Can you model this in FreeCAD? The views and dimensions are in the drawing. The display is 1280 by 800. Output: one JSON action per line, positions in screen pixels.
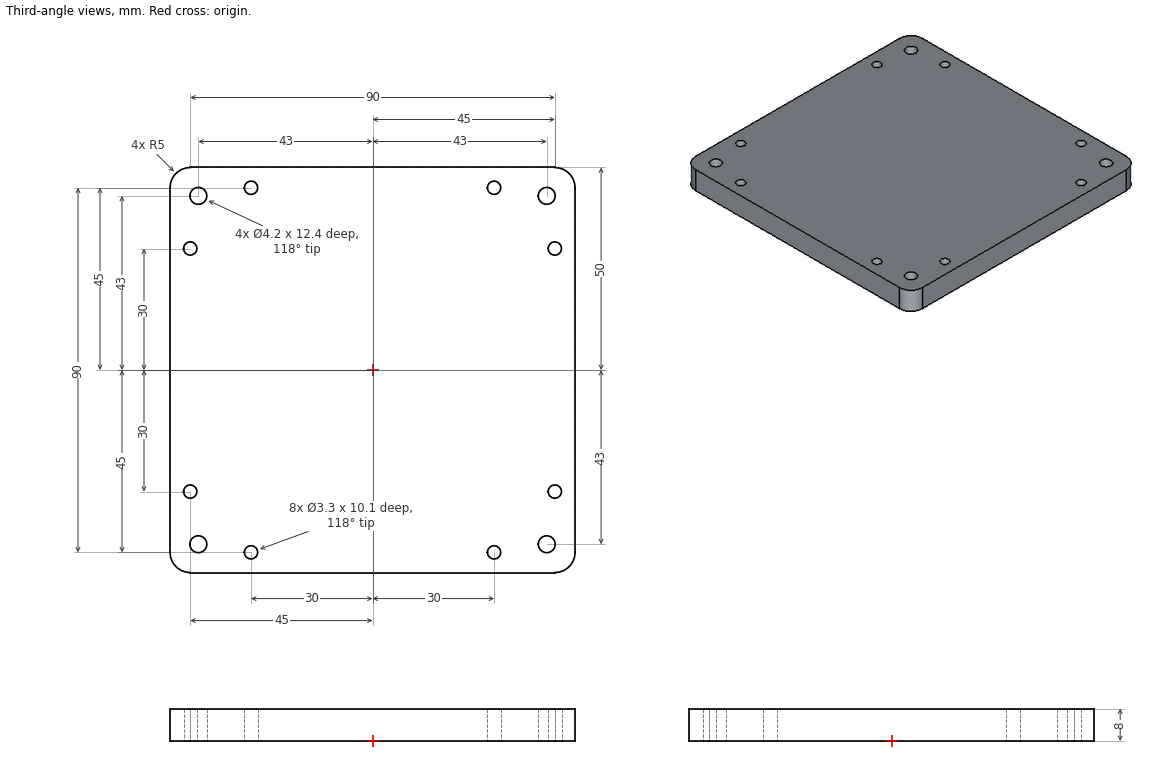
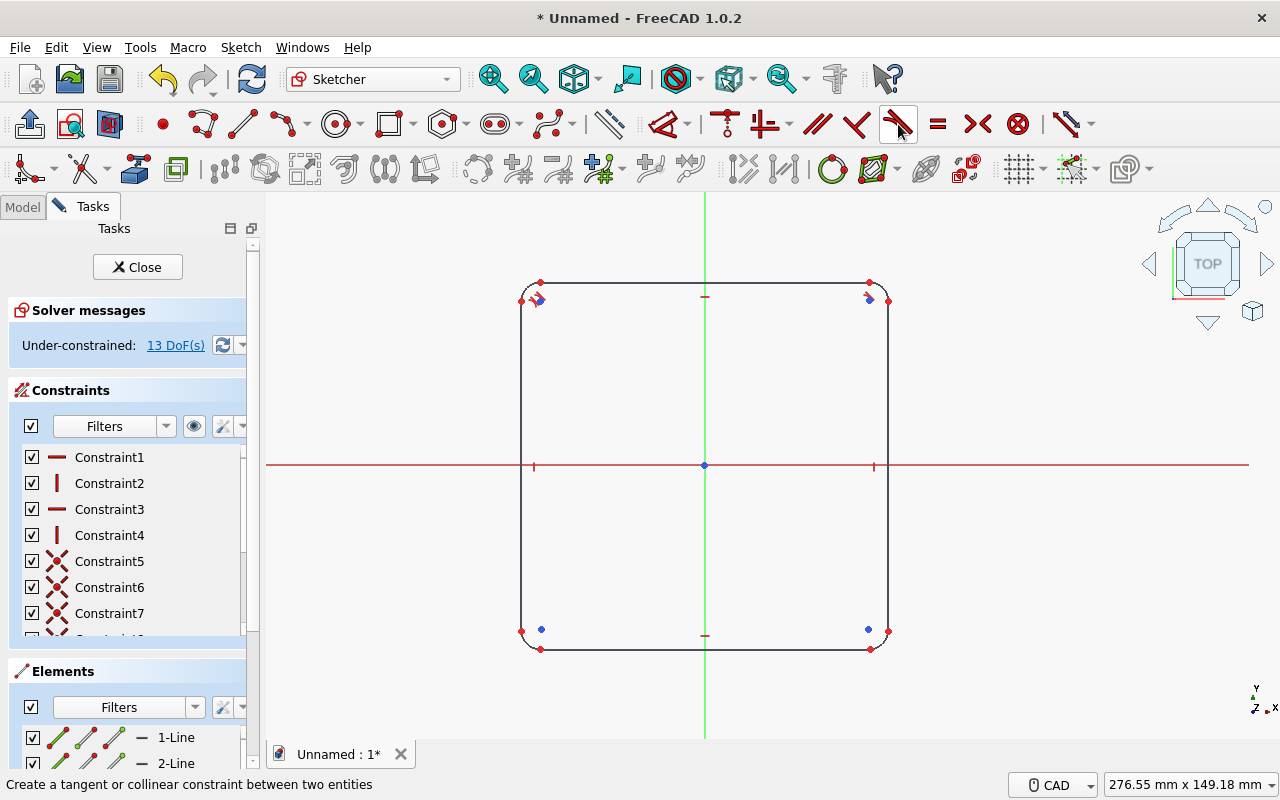
{"action": "left_click", "coordinate": [521, 401]}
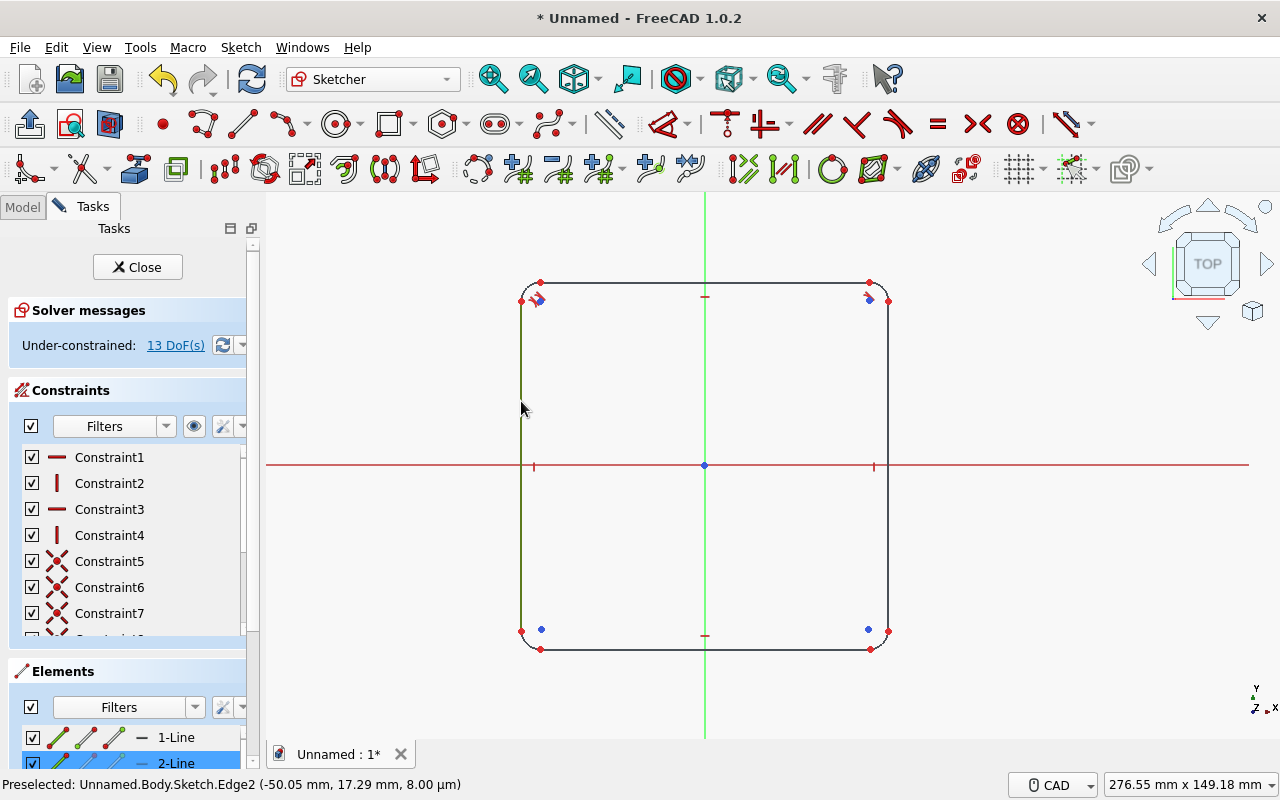
{"action": "left_click", "coordinate": [527, 644]}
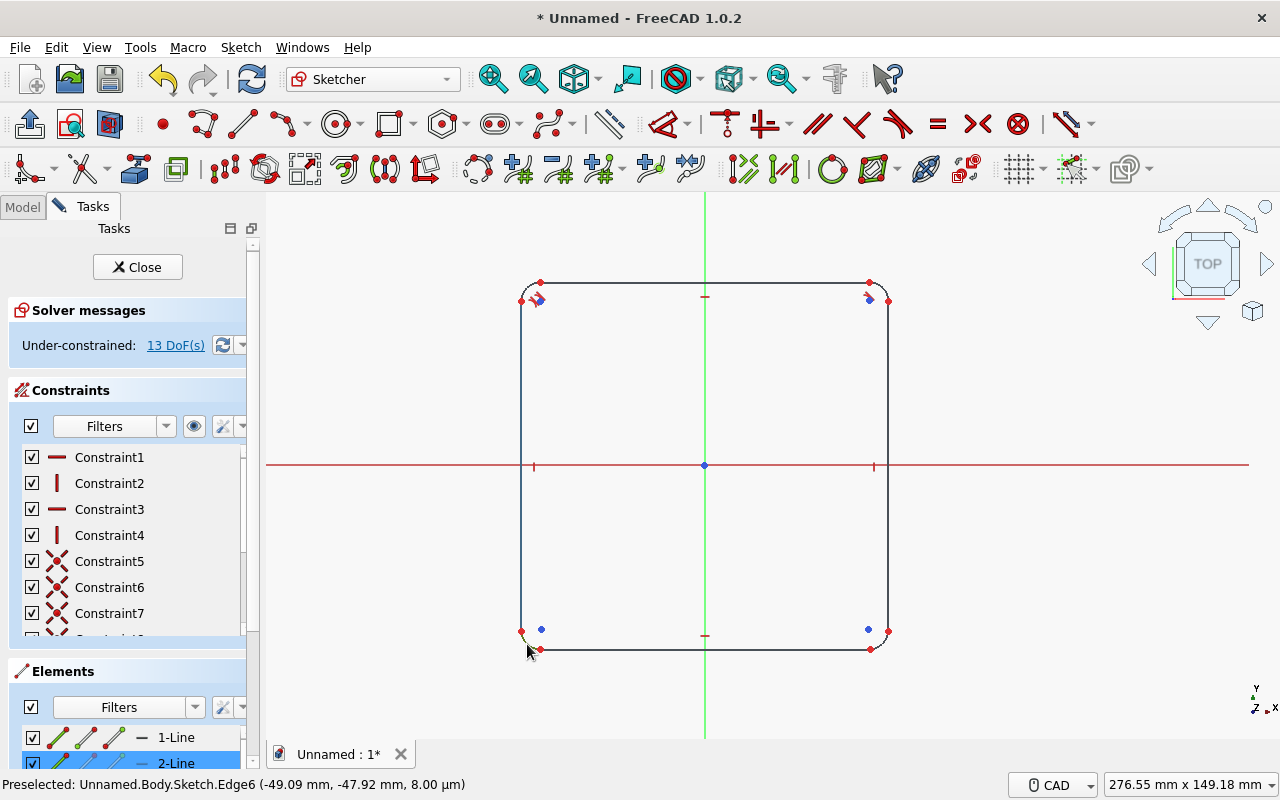
{"action": "key", "text": "t"}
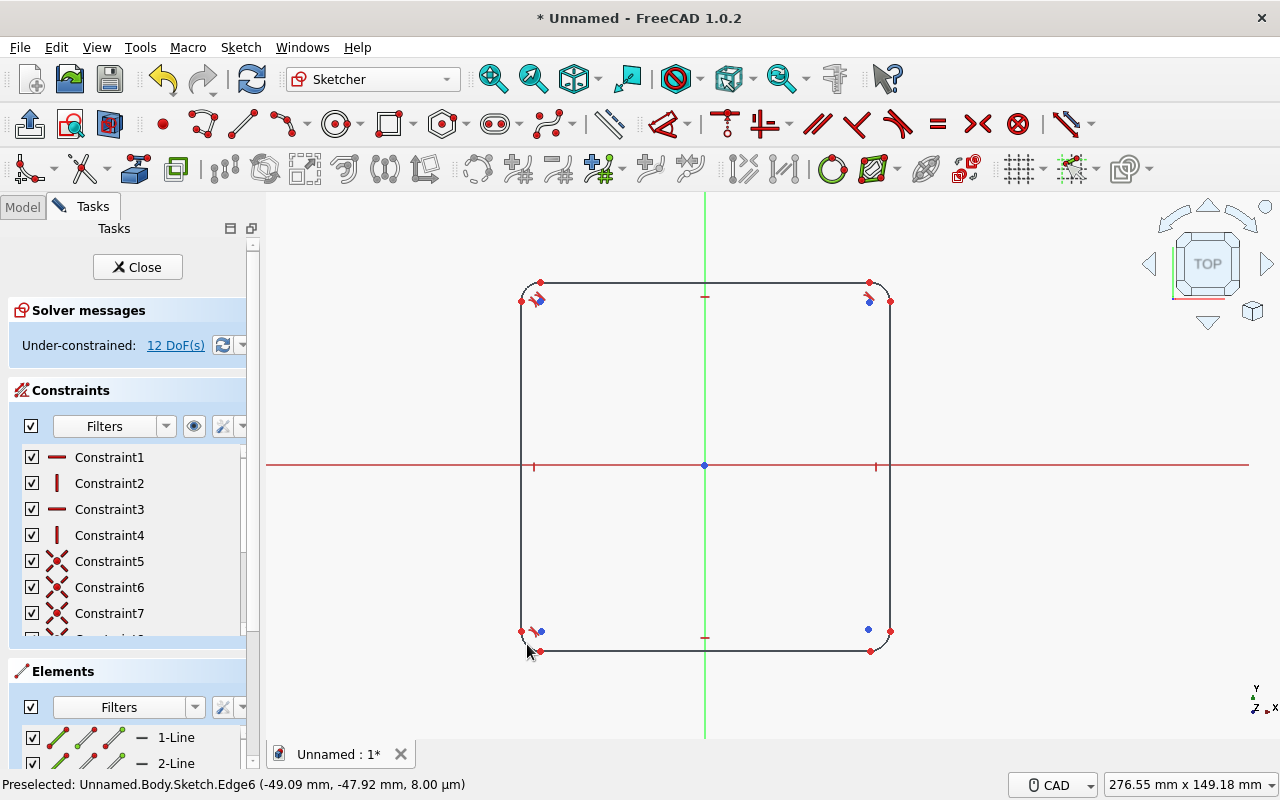
{"action": "left_click", "coordinate": [639, 651]}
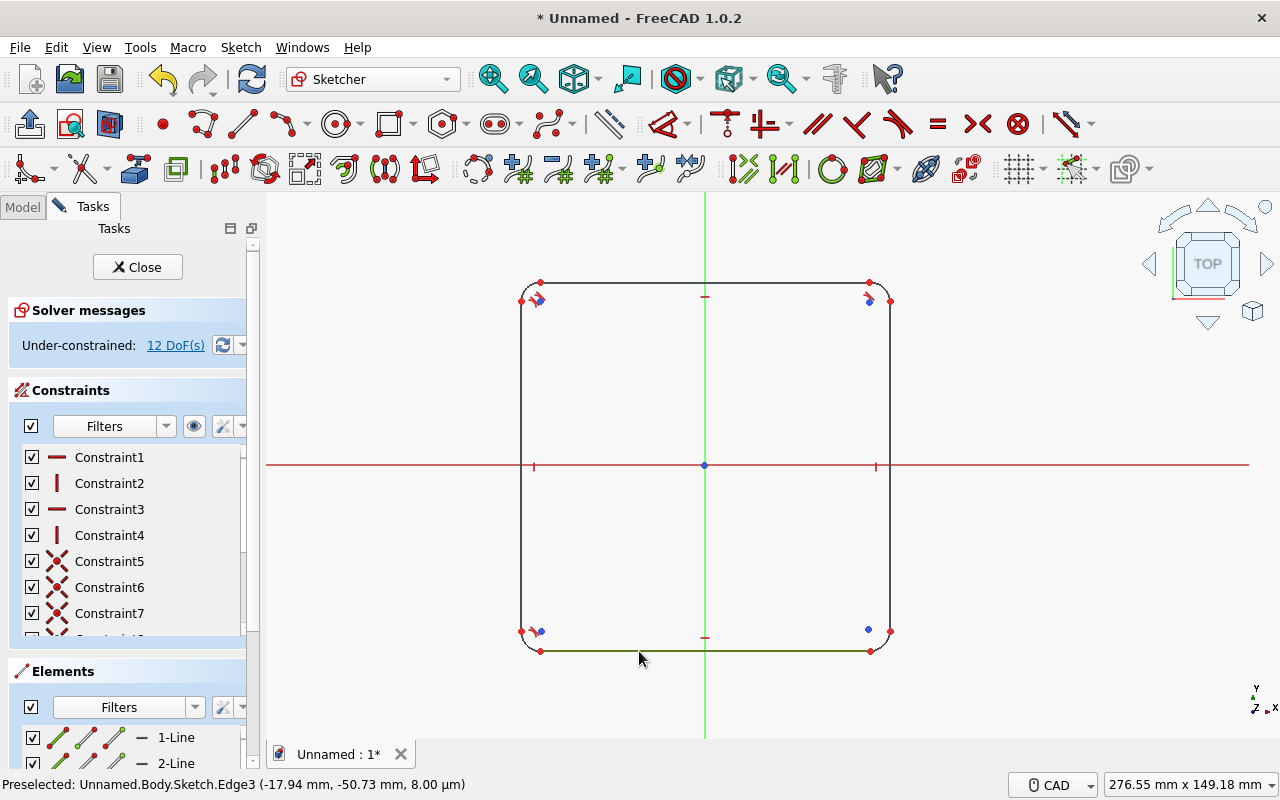
{"action": "scroll", "coordinate": [523, 640], "scroll_direction": "up", "scroll_amount": 3}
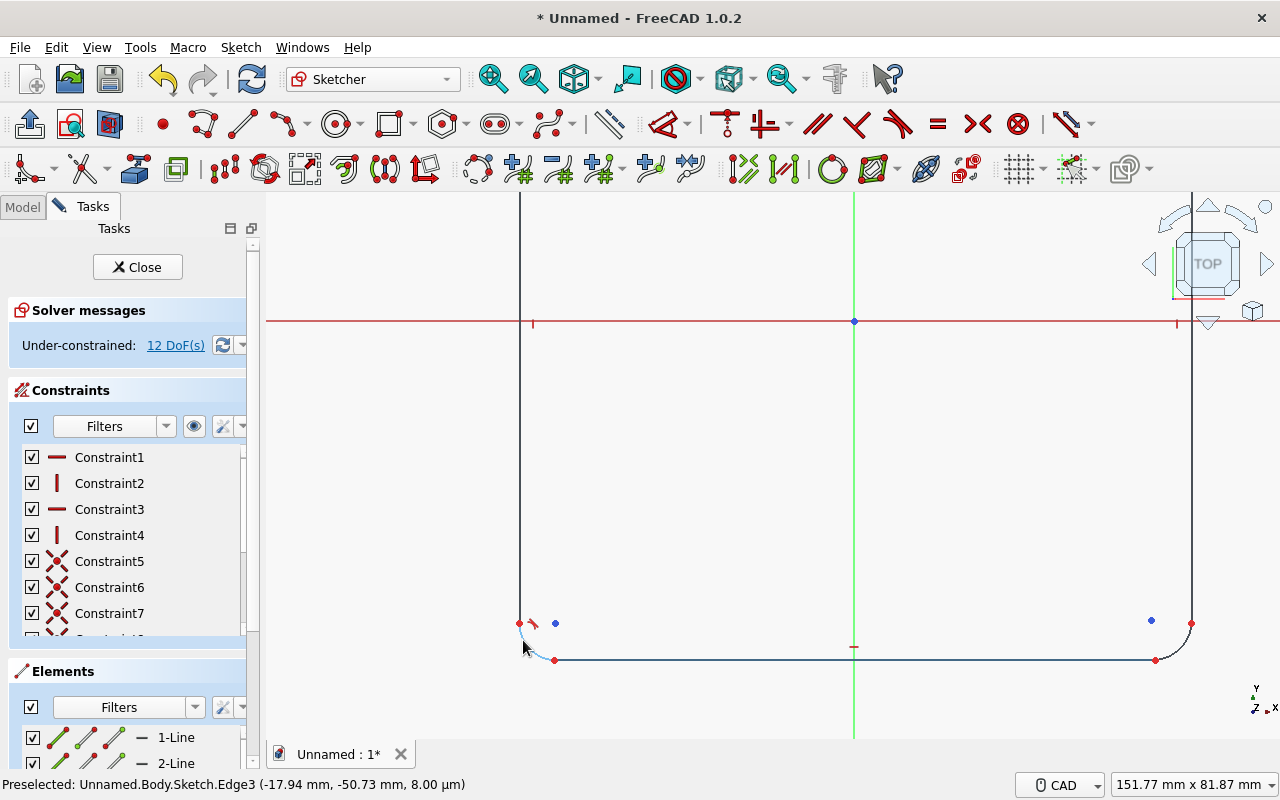
{"action": "left_click", "coordinate": [523, 640]}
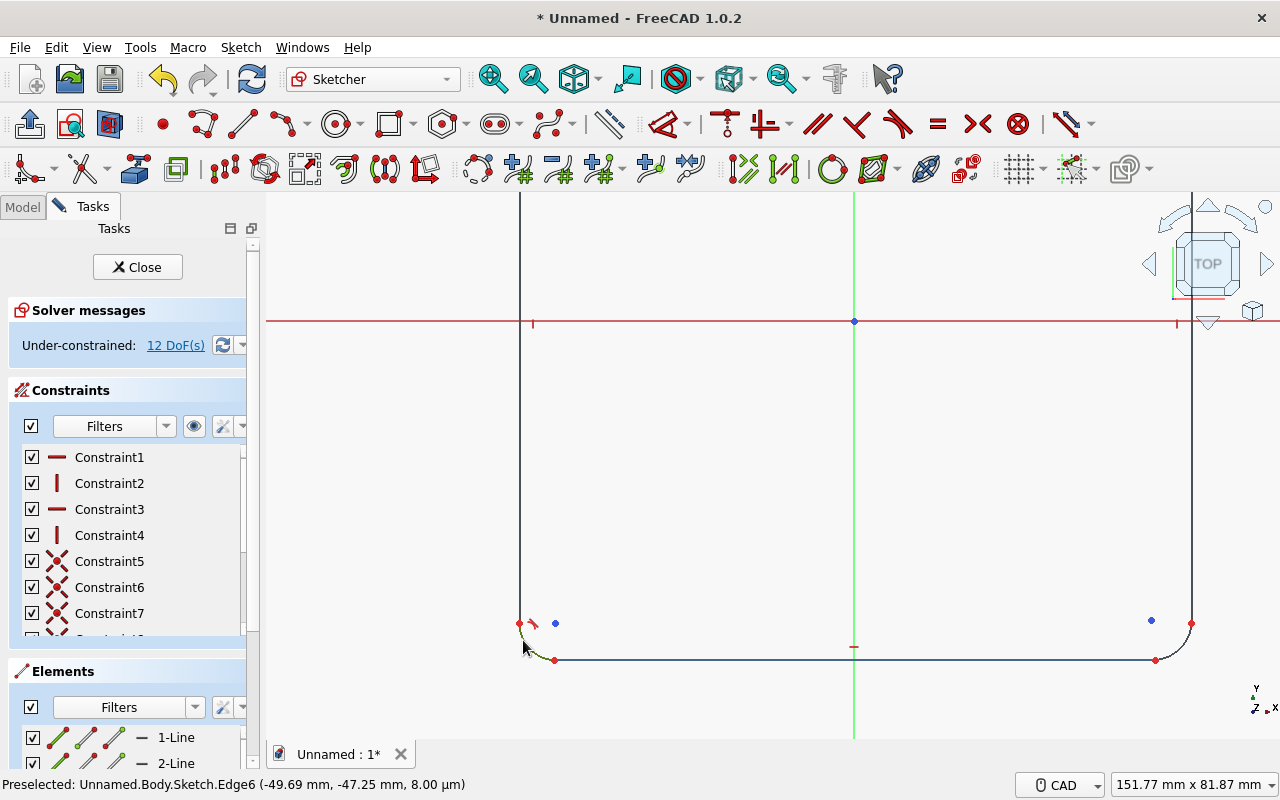
{"action": "key", "text": "t"}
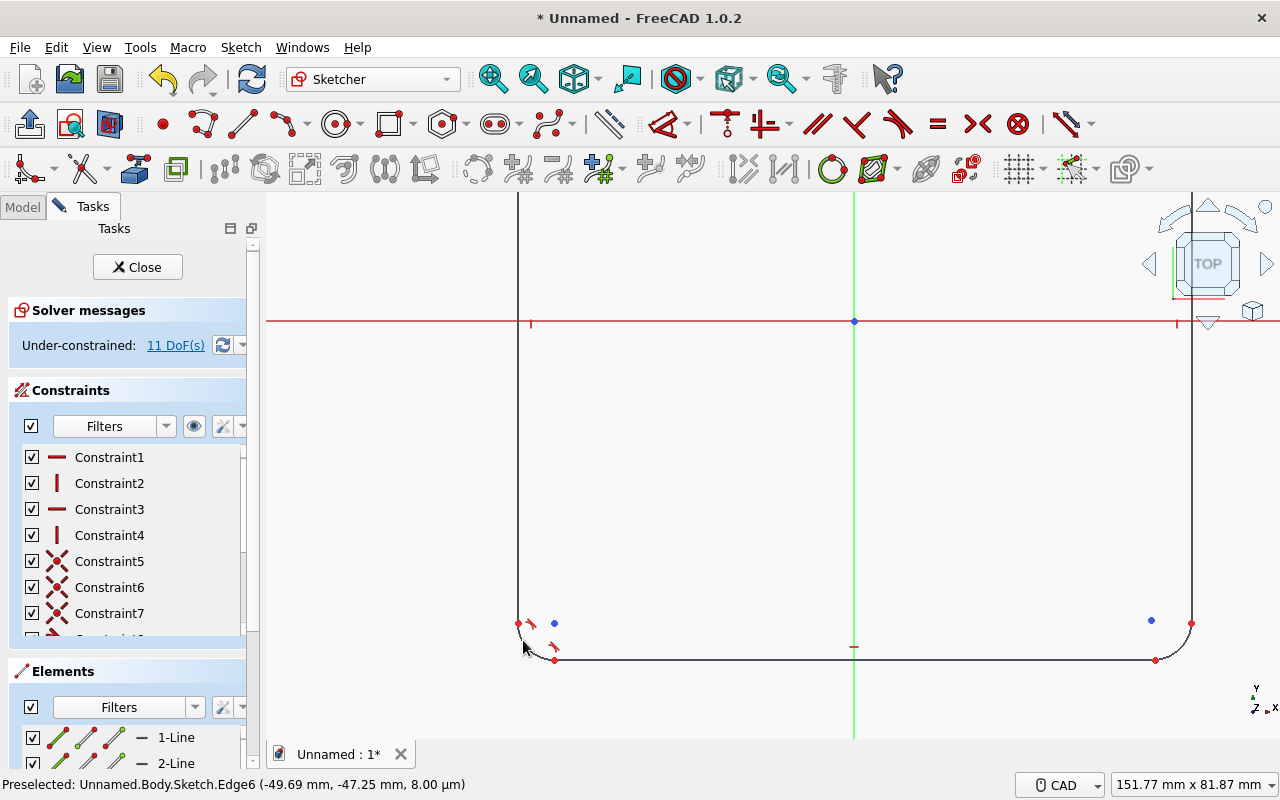
{"action": "left_click", "coordinate": [735, 660]}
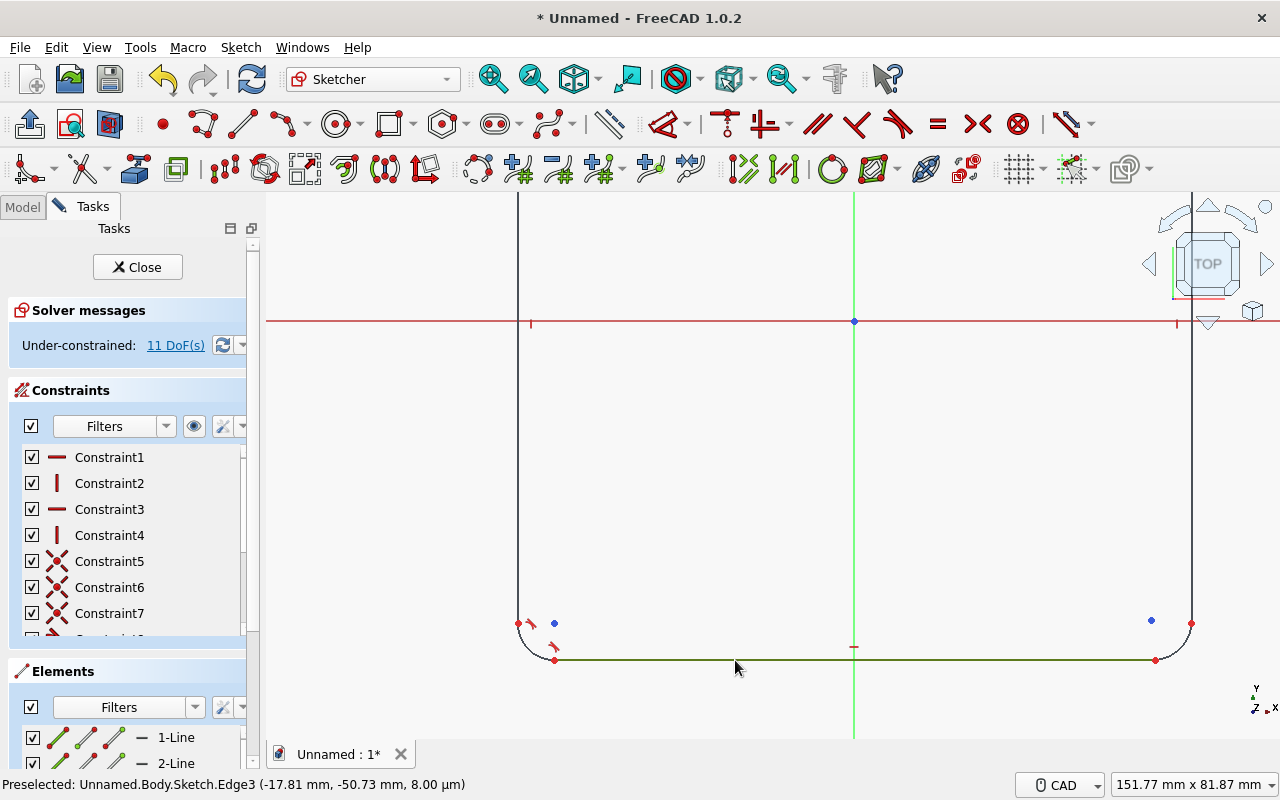
{"action": "scroll", "coordinate": [523, 641], "scroll_direction": "down", "scroll_amount": 3}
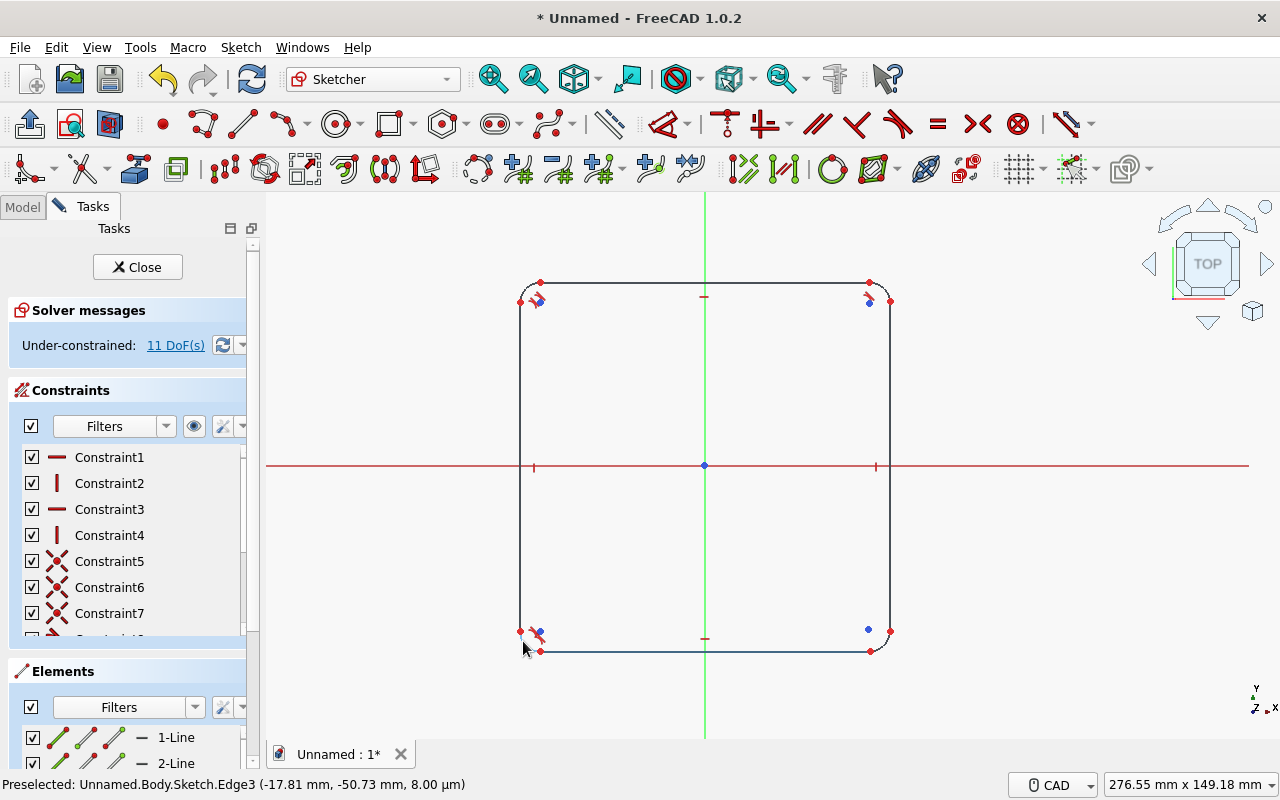
{"action": "scroll", "coordinate": [879, 649], "scroll_direction": "up", "scroll_amount": 3}